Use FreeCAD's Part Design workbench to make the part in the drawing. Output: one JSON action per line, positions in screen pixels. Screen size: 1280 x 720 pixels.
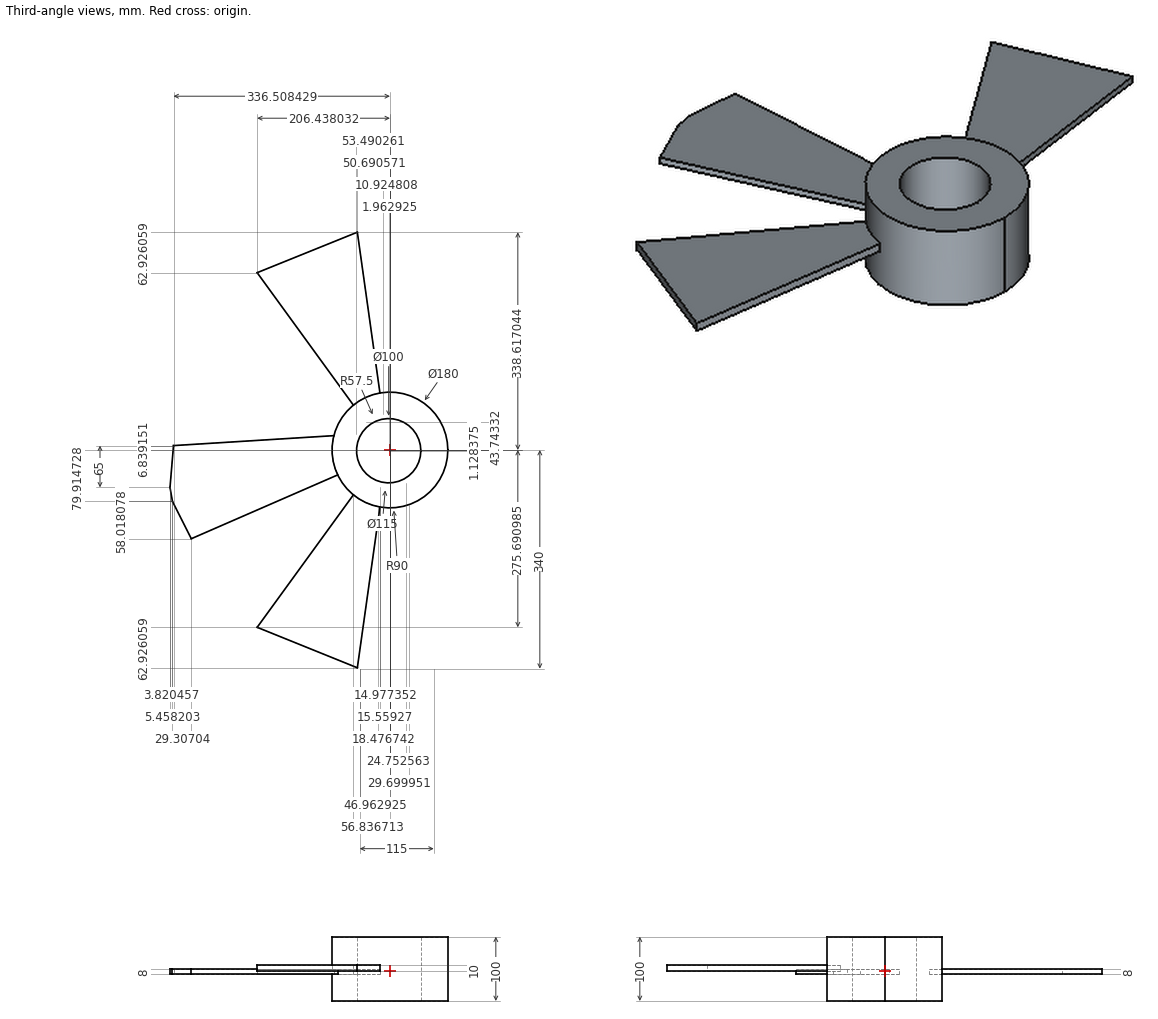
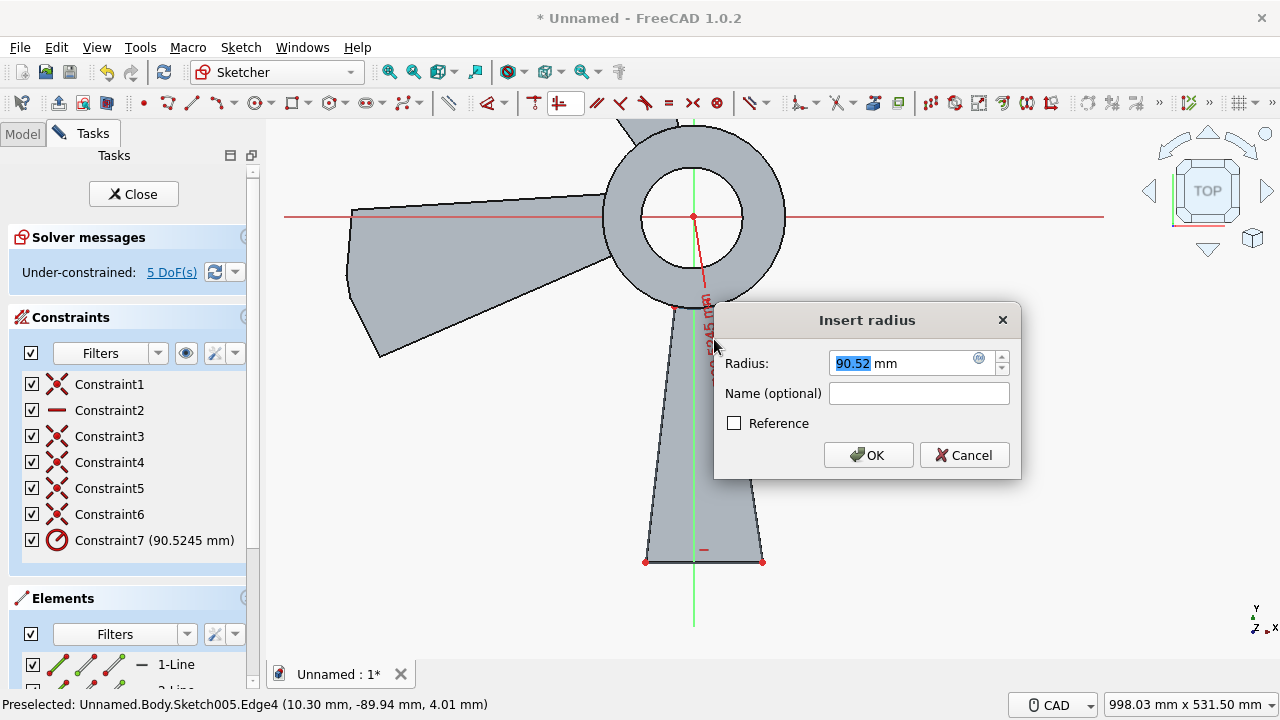
{"action": "type", "text": "90"}
{"action": "key", "text": "Return"}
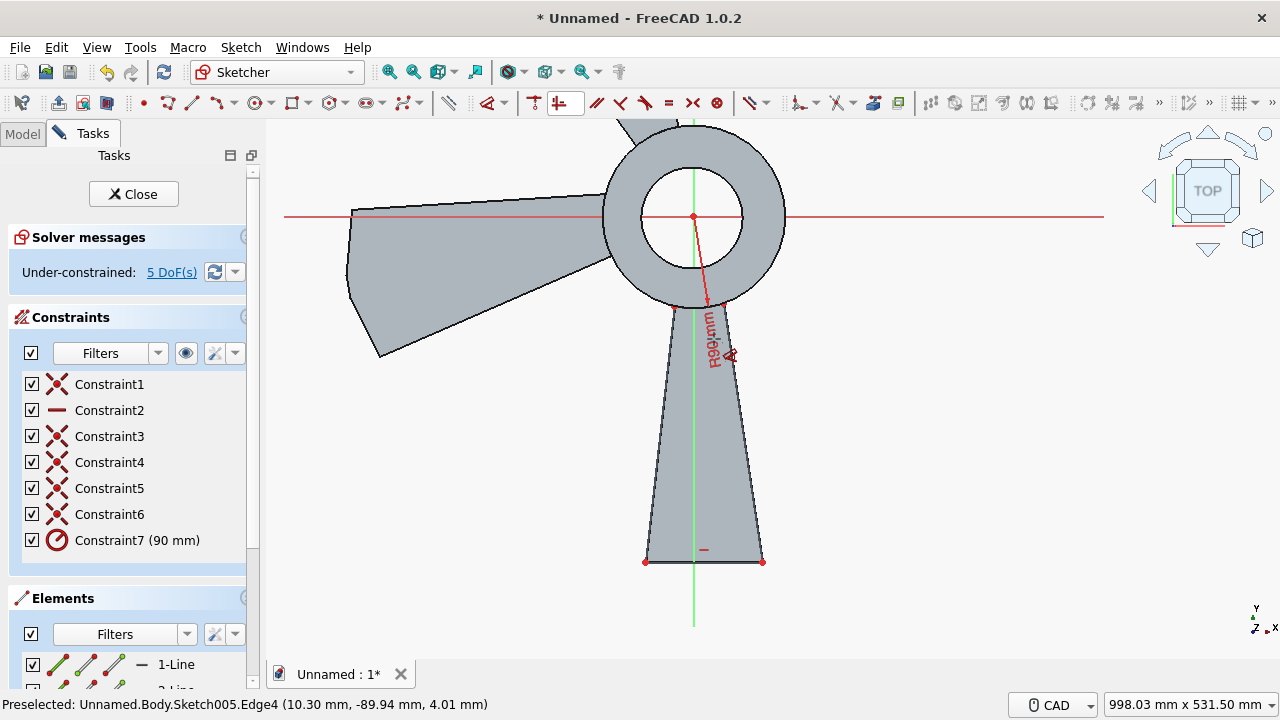
{"action": "left_click", "coordinate": [681, 563]}
{"action": "left_click", "coordinate": [677, 597]}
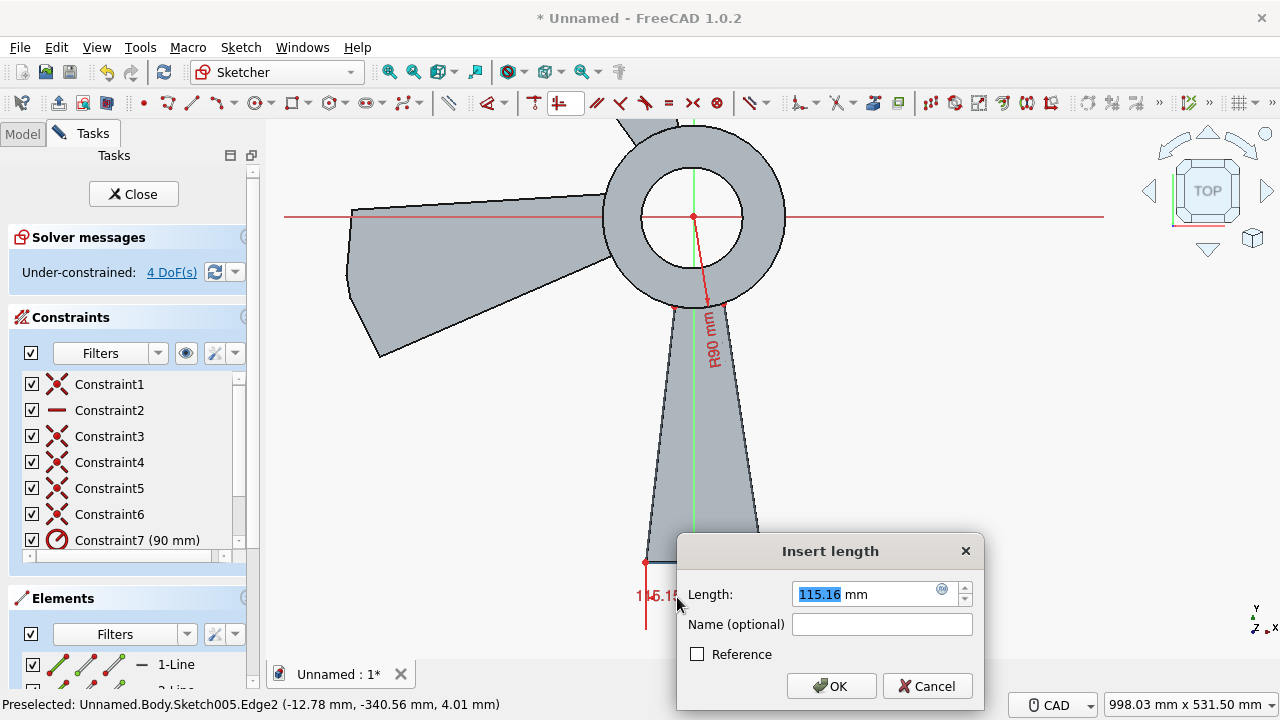
{"action": "type", "text": "115"}
{"action": "key", "text": "Return"}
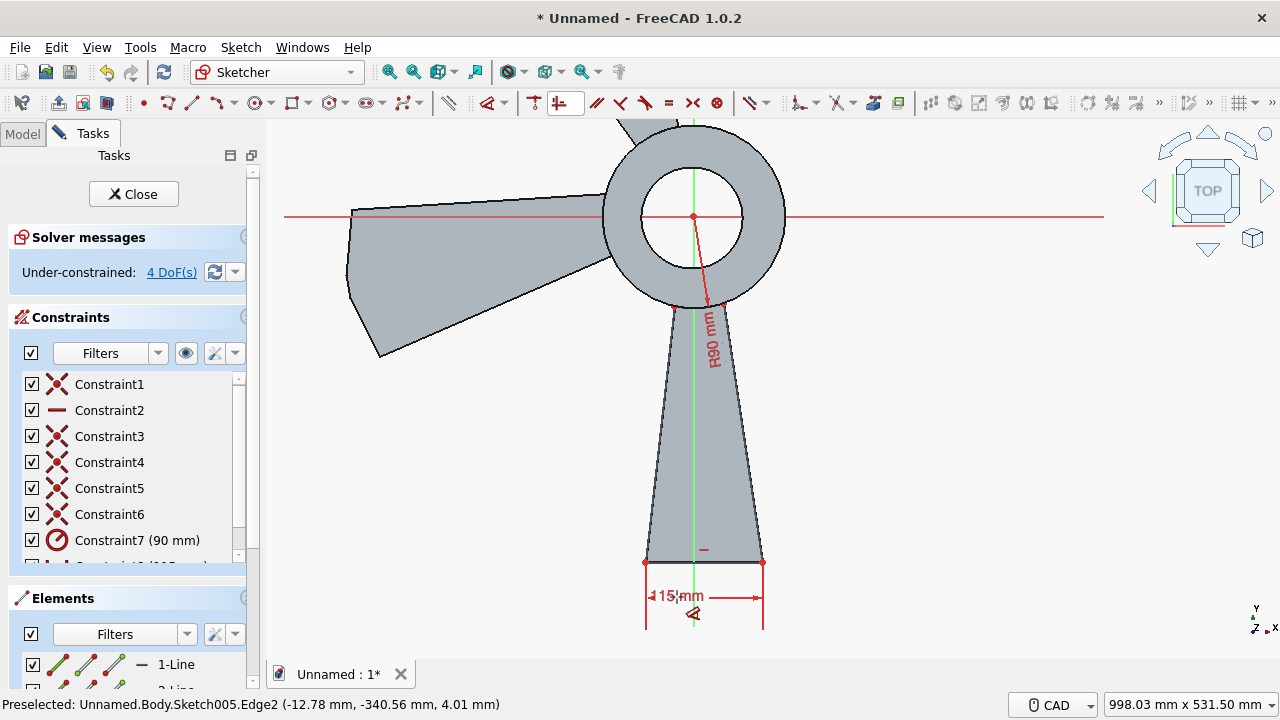
{"action": "left_click", "coordinate": [646, 563]}
{"action": "left_click", "coordinate": [612, 390]}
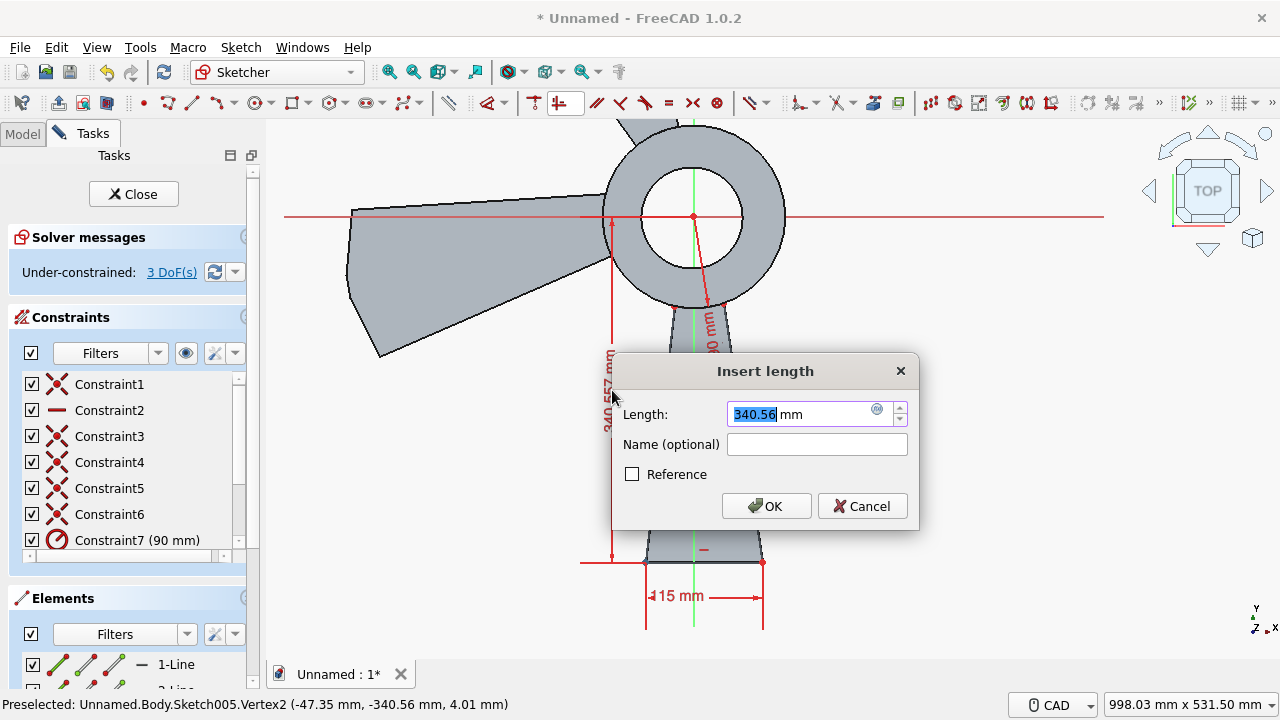
{"action": "type", "text": "340"}
{"action": "key", "text": "Return"}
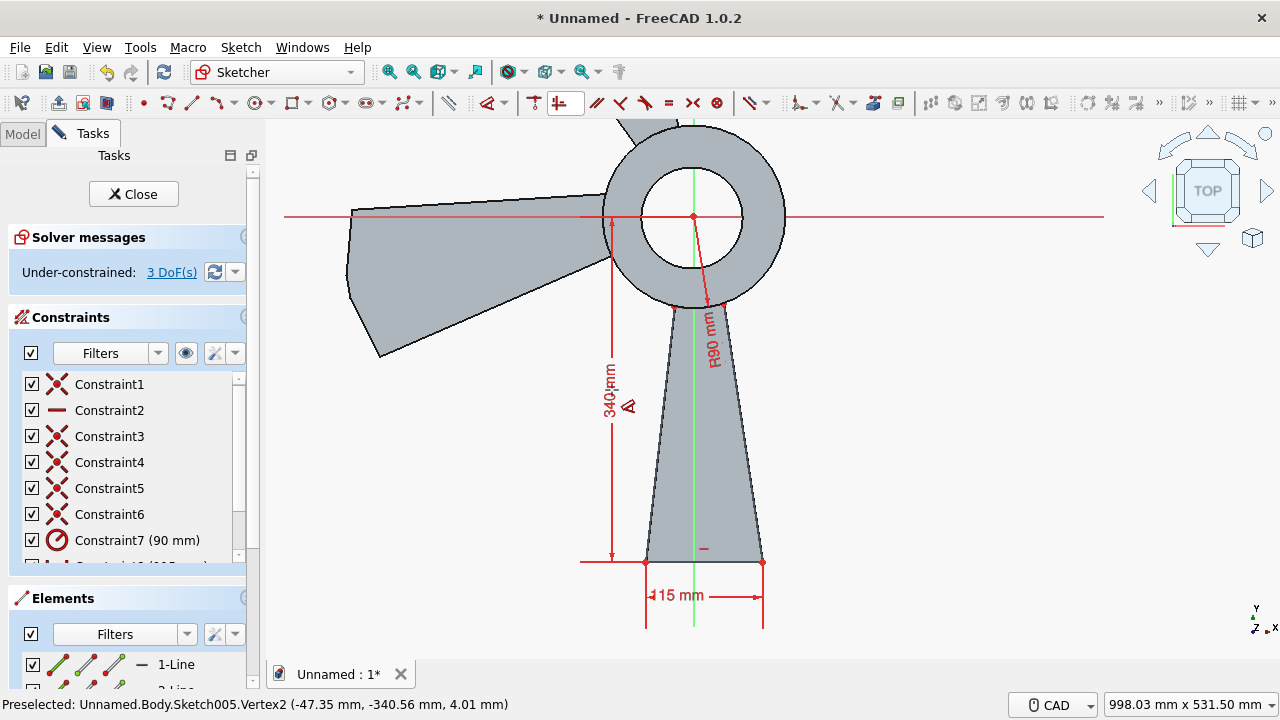
{"action": "scroll", "coordinate": [675, 306], "scroll_direction": "up", "scroll_amount": 4}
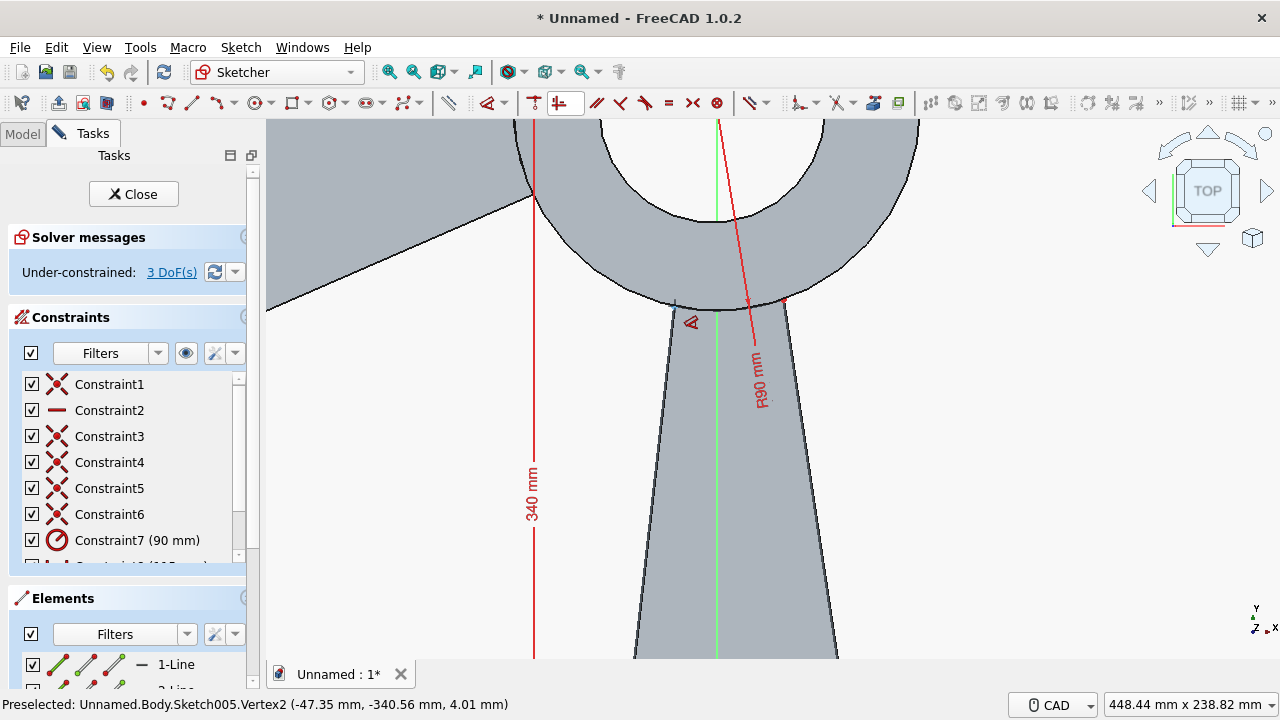
{"action": "left_click", "coordinate": [674, 306]}
{"action": "left_click", "coordinate": [695, 340]}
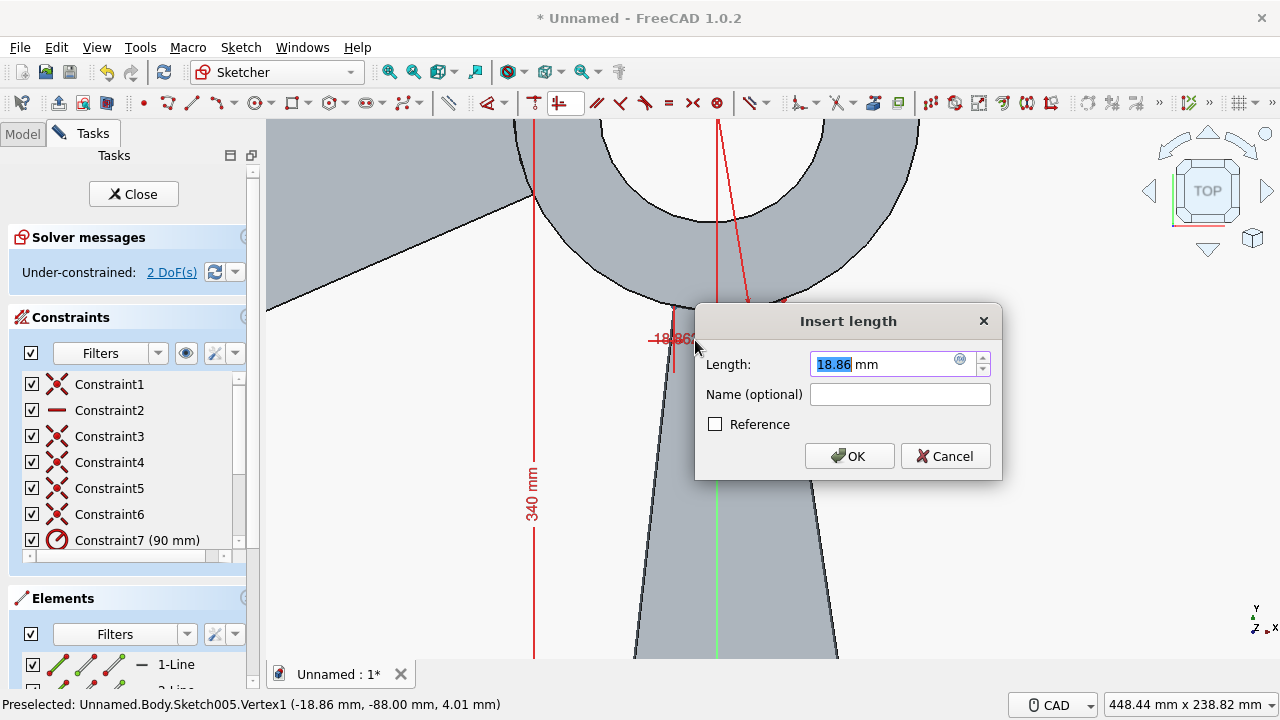
{"action": "type", "text": "18.476742"}
{"action": "key", "text": "Return"}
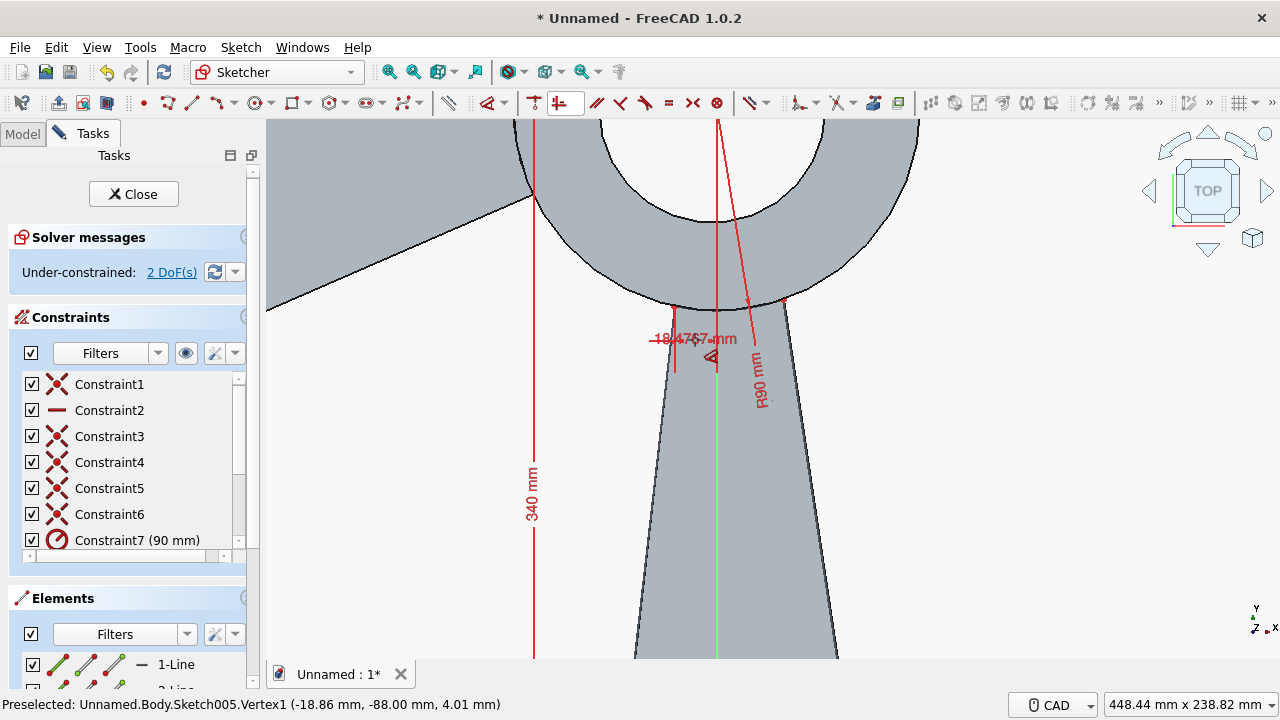
{"action": "scroll", "coordinate": [675, 305], "scroll_direction": "down", "scroll_amount": 4}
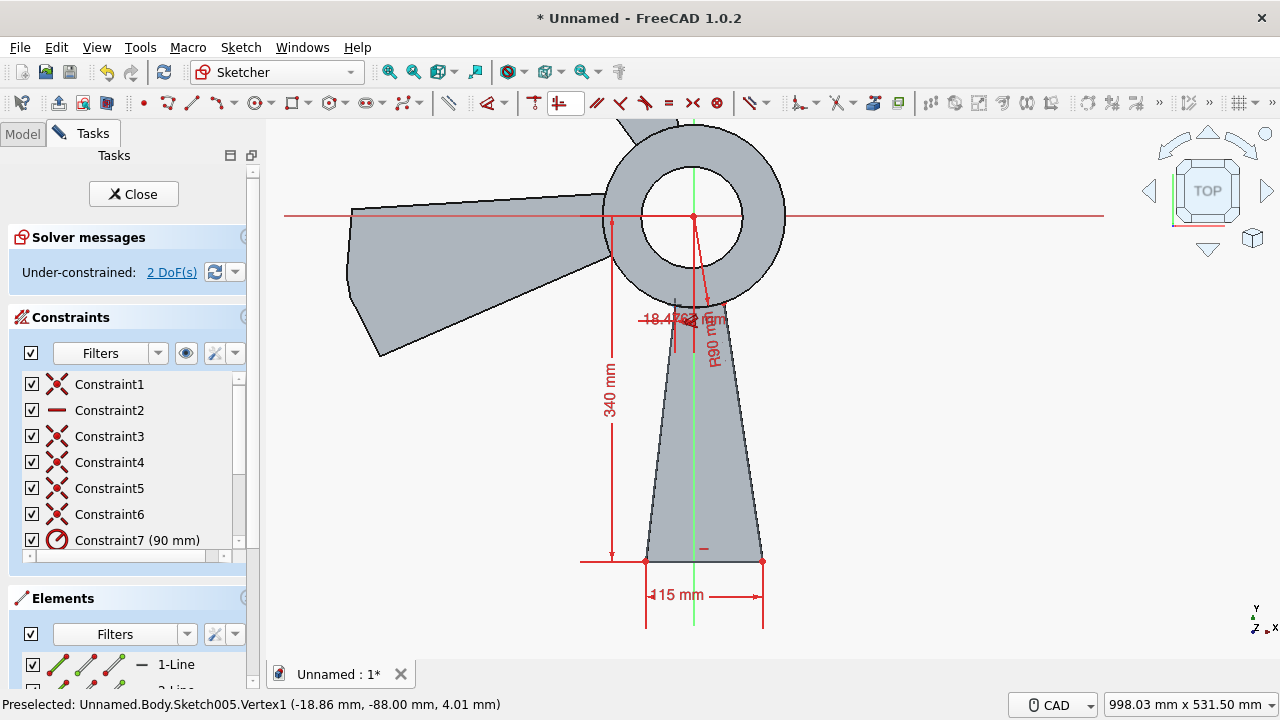
{"action": "left_click", "coordinate": [646, 562]}
{"action": "left_click", "coordinate": [670, 182]}